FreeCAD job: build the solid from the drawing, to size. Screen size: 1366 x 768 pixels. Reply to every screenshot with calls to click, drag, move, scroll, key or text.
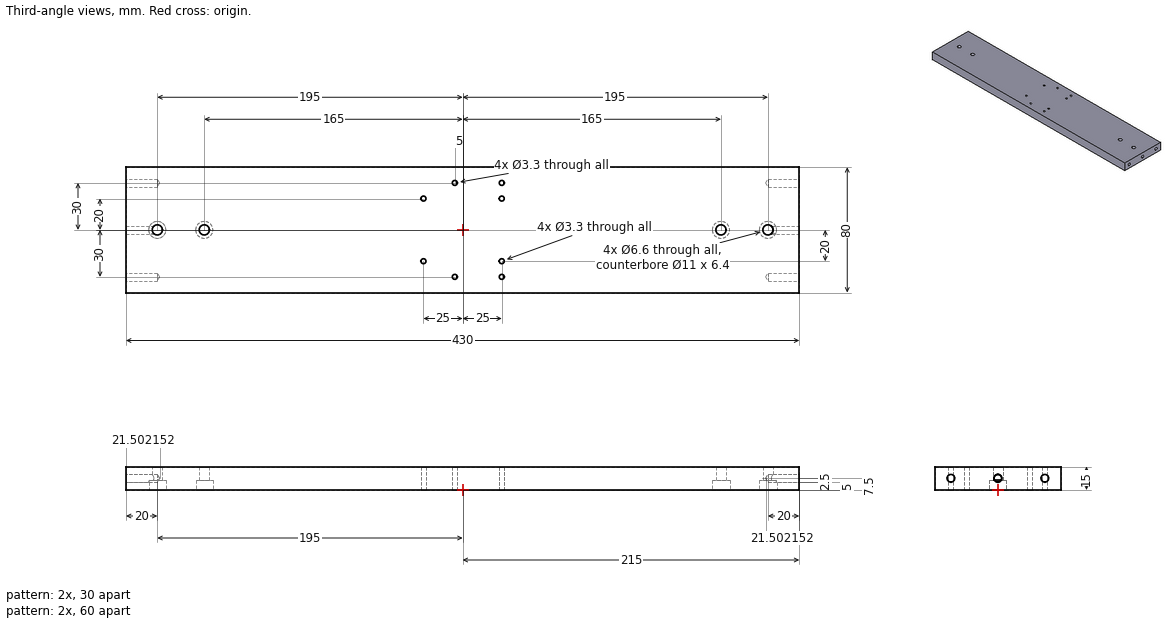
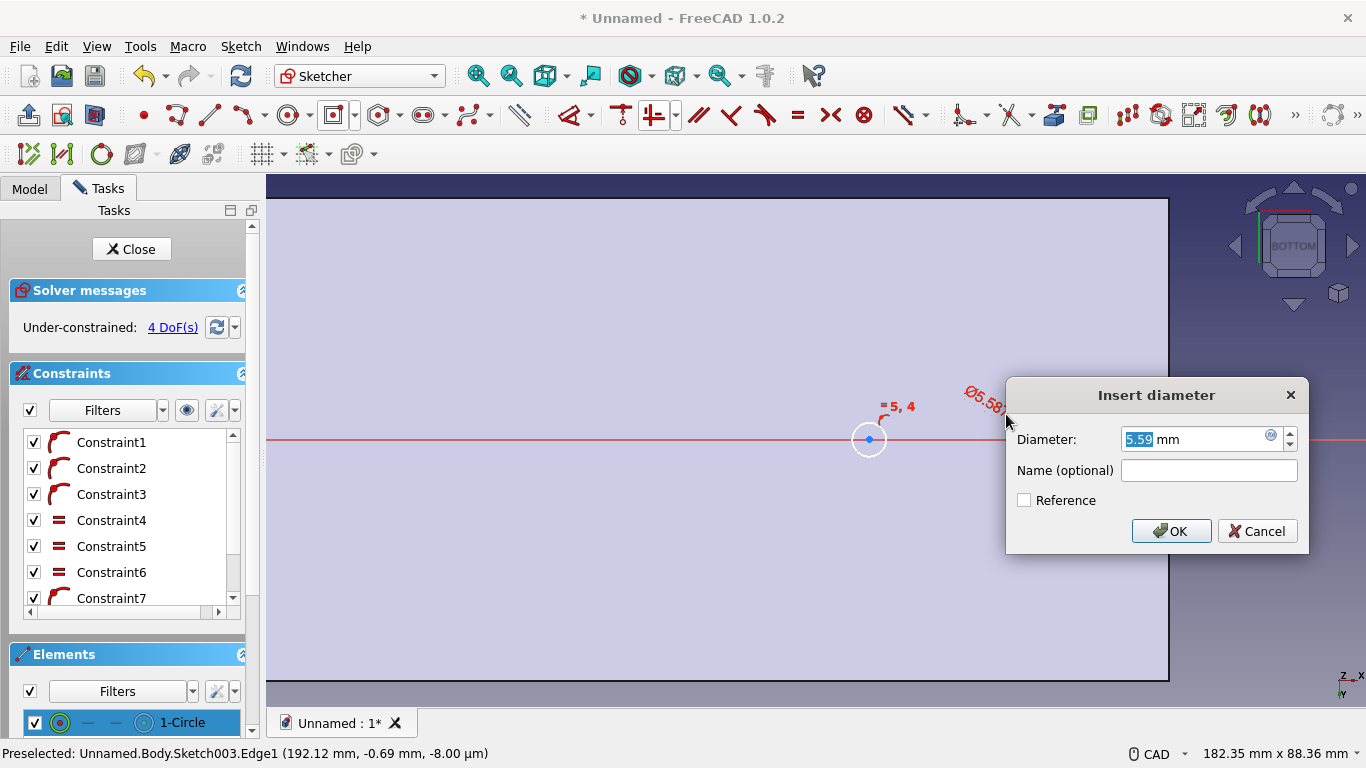
text(6.6)
key(Return)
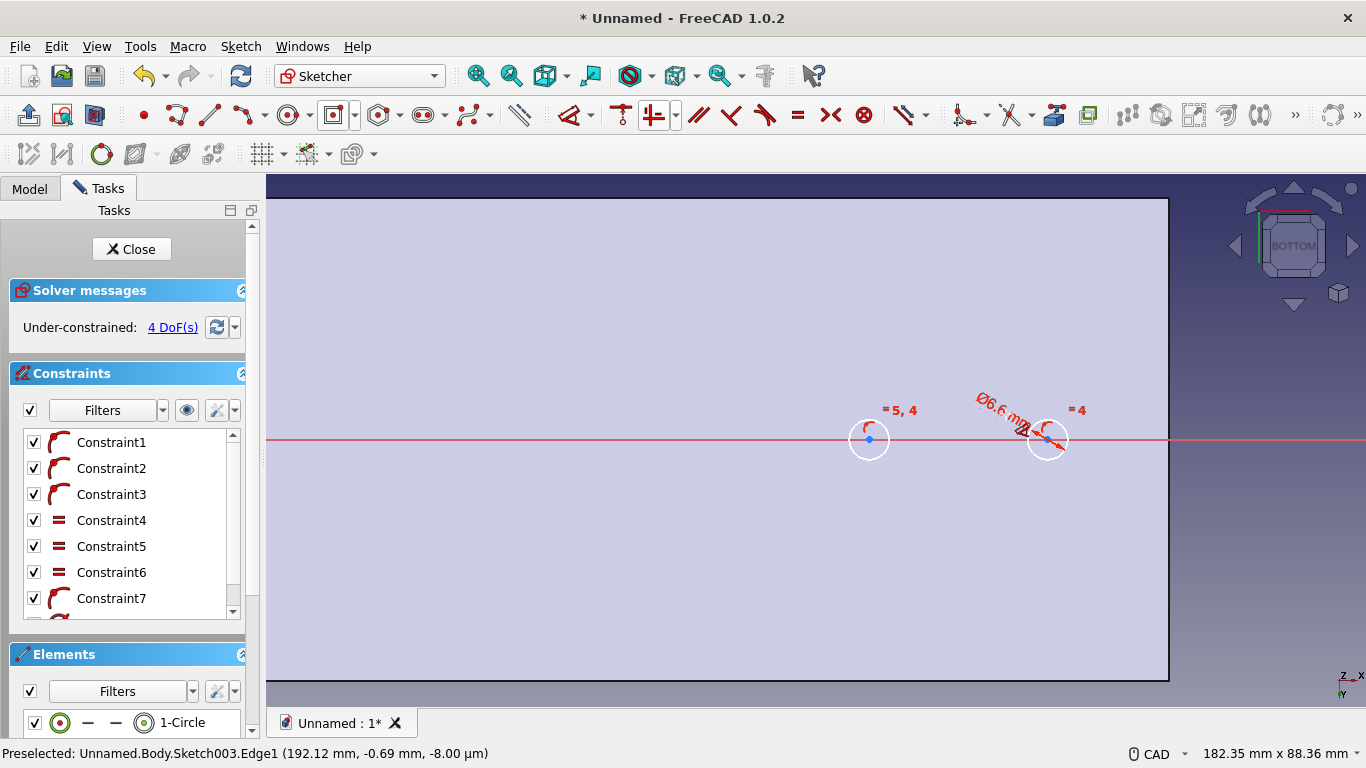
scroll(1034, 441, down, 7)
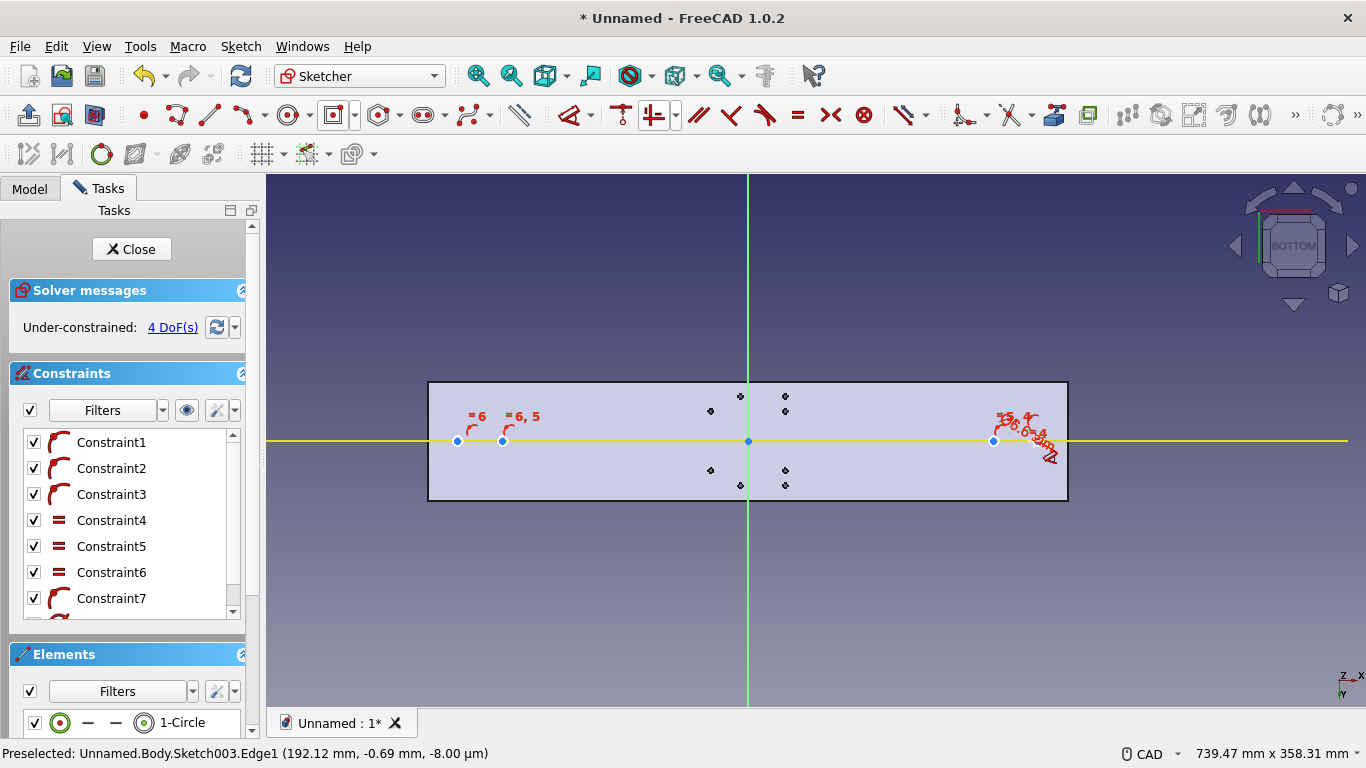
click(1038, 441)
click(893, 475)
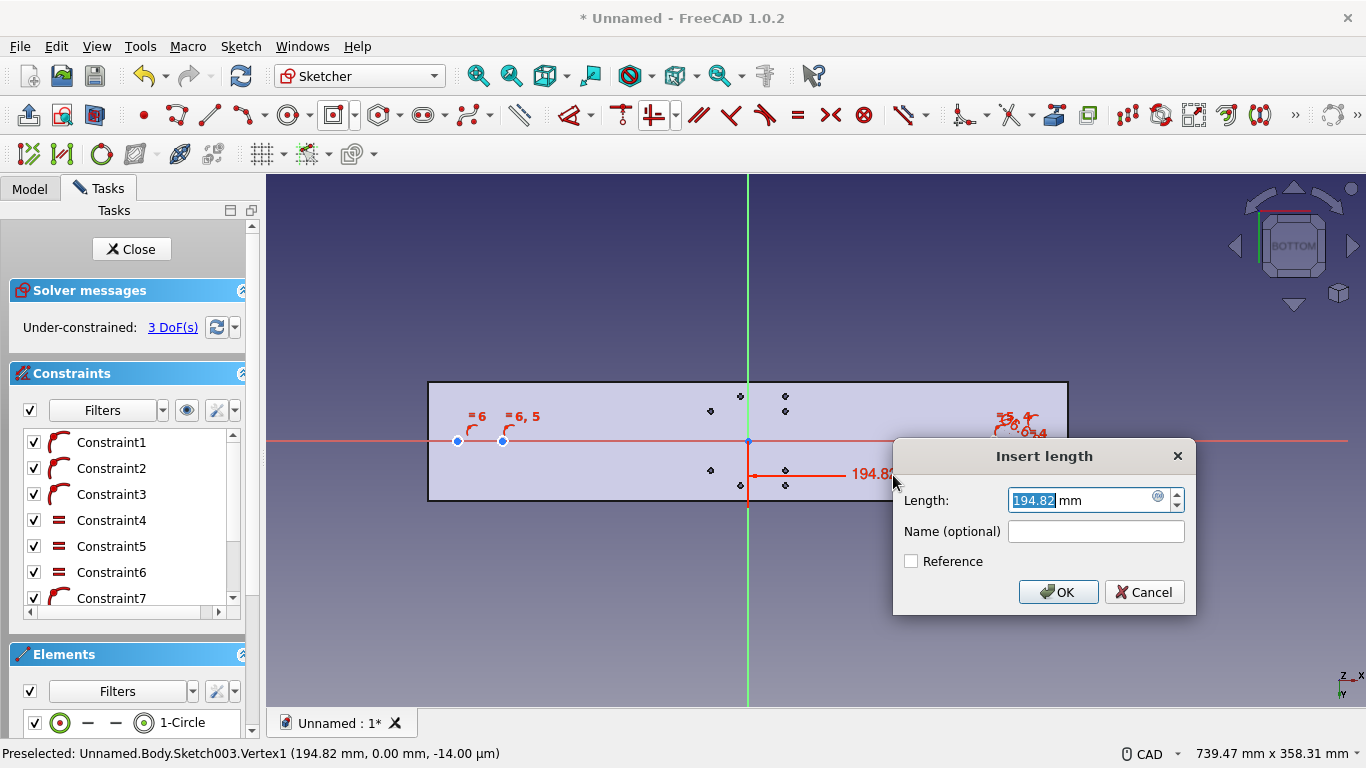
text(195)
key(Return)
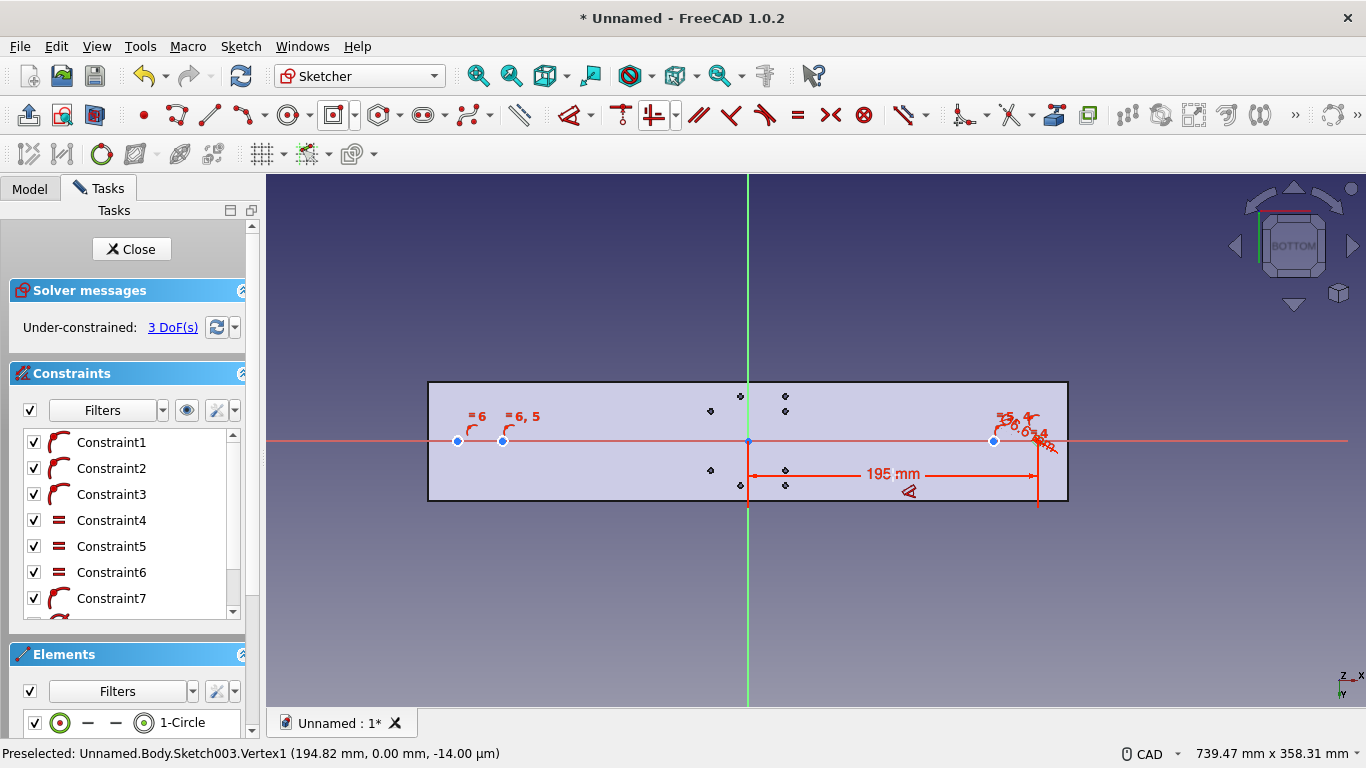
click(994, 441)
click(814, 475)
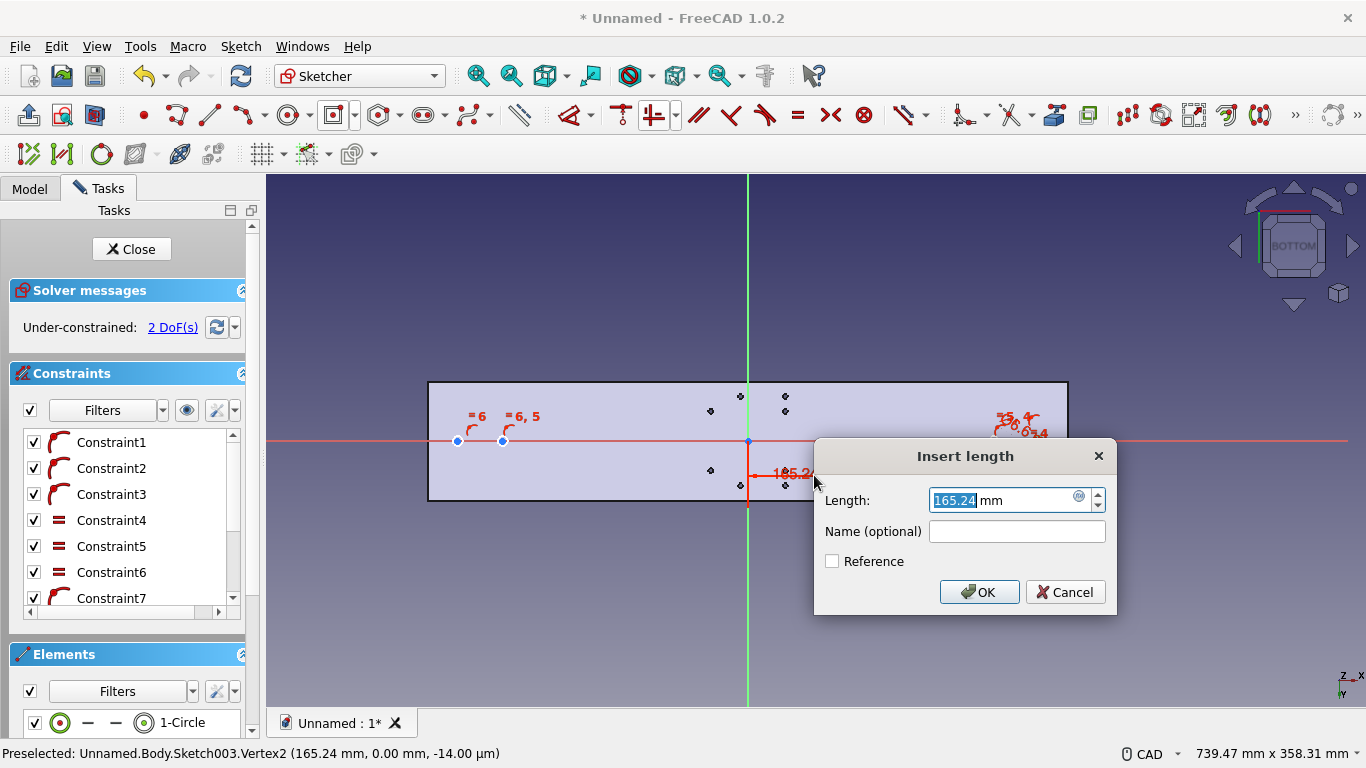
text(165)
key(Return)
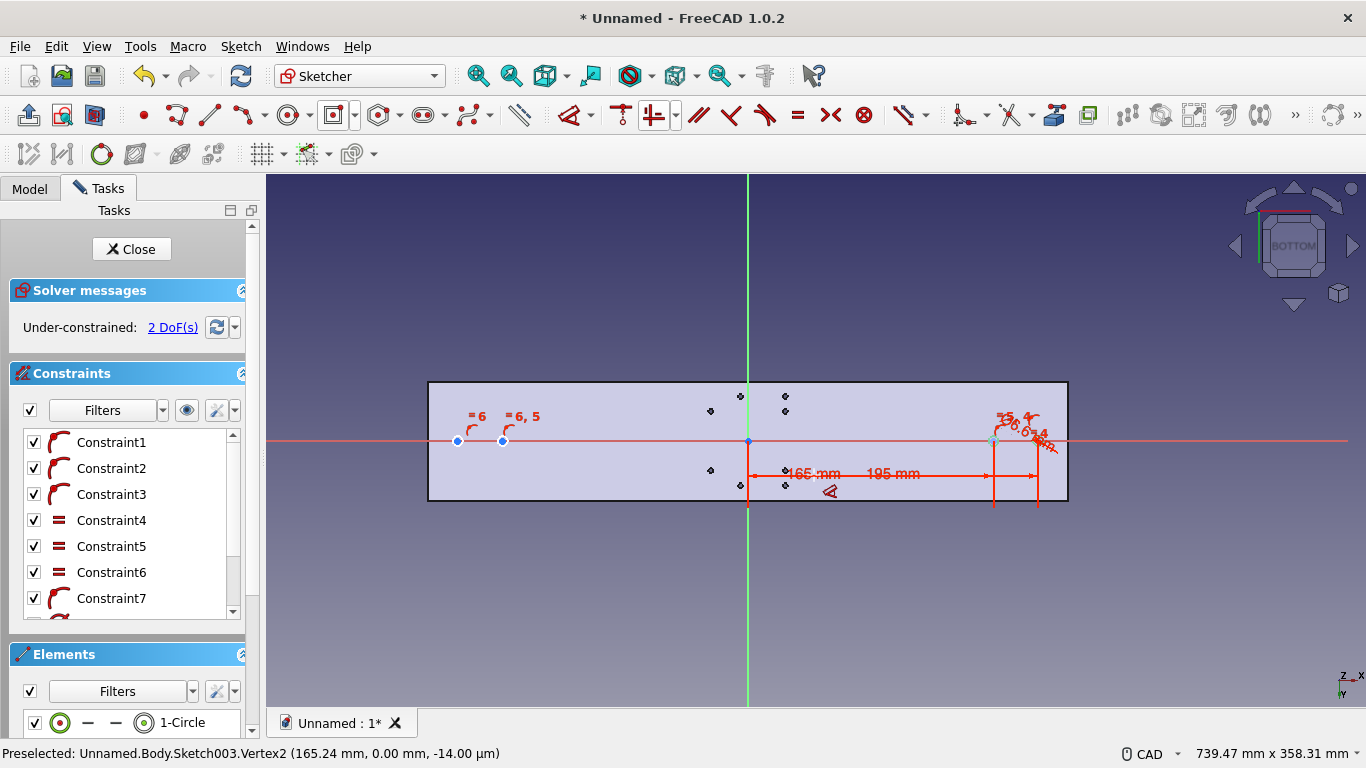
click(503, 441)
click(625, 475)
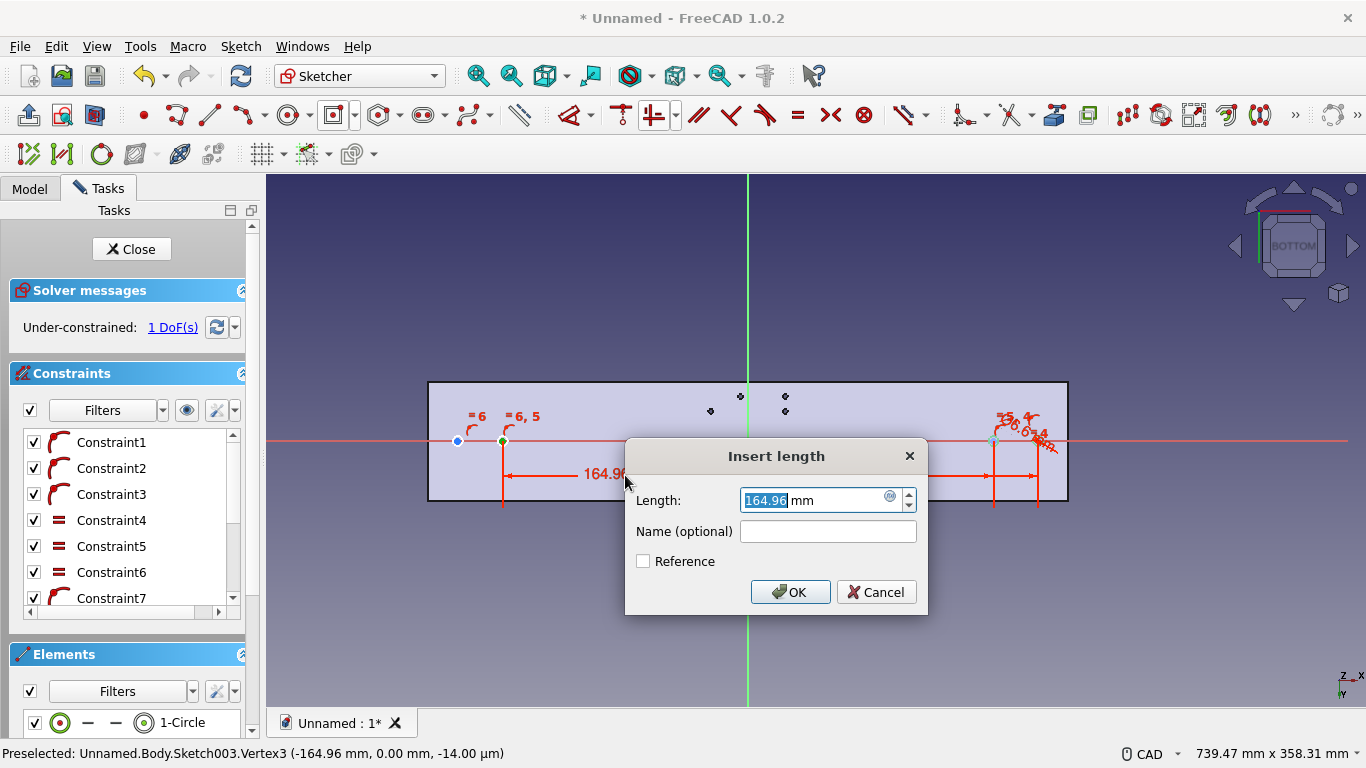
text(165)
key(Return)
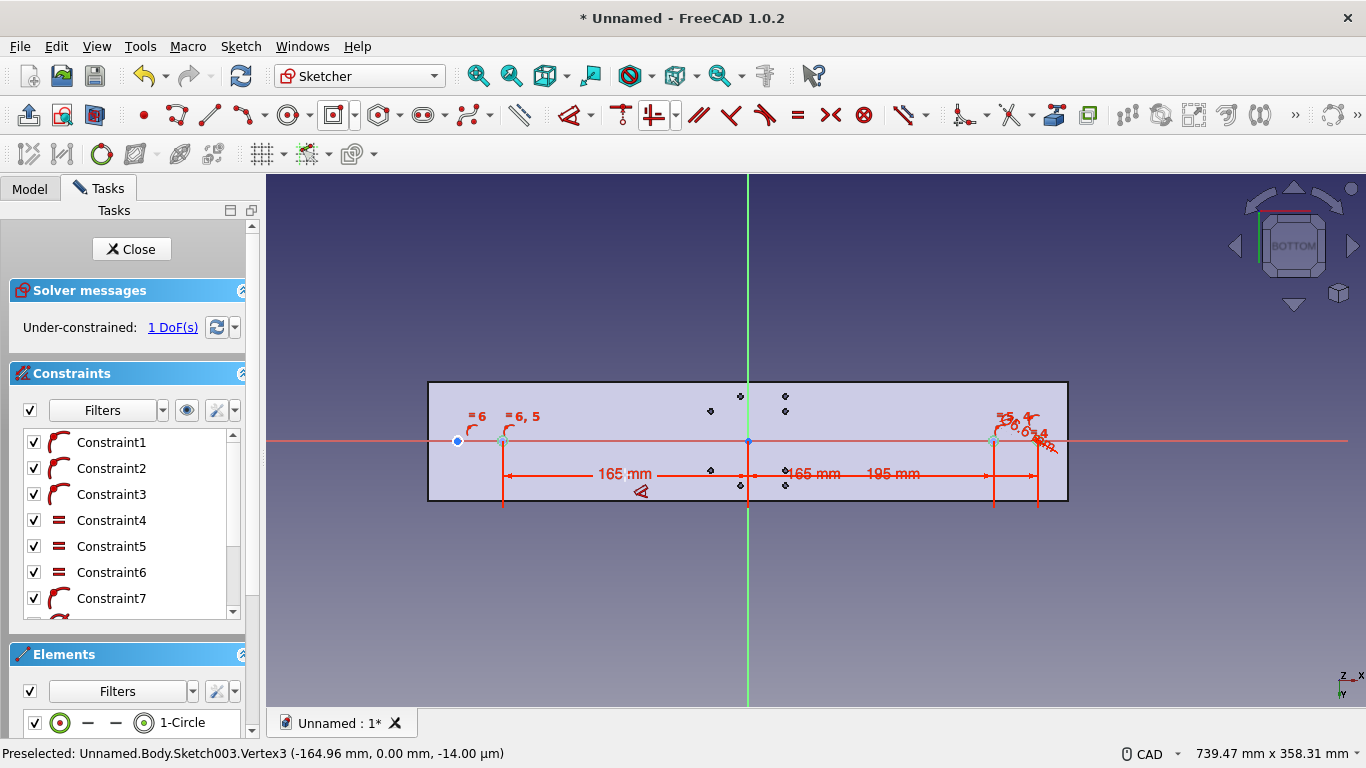
click(458, 441)
click(536, 475)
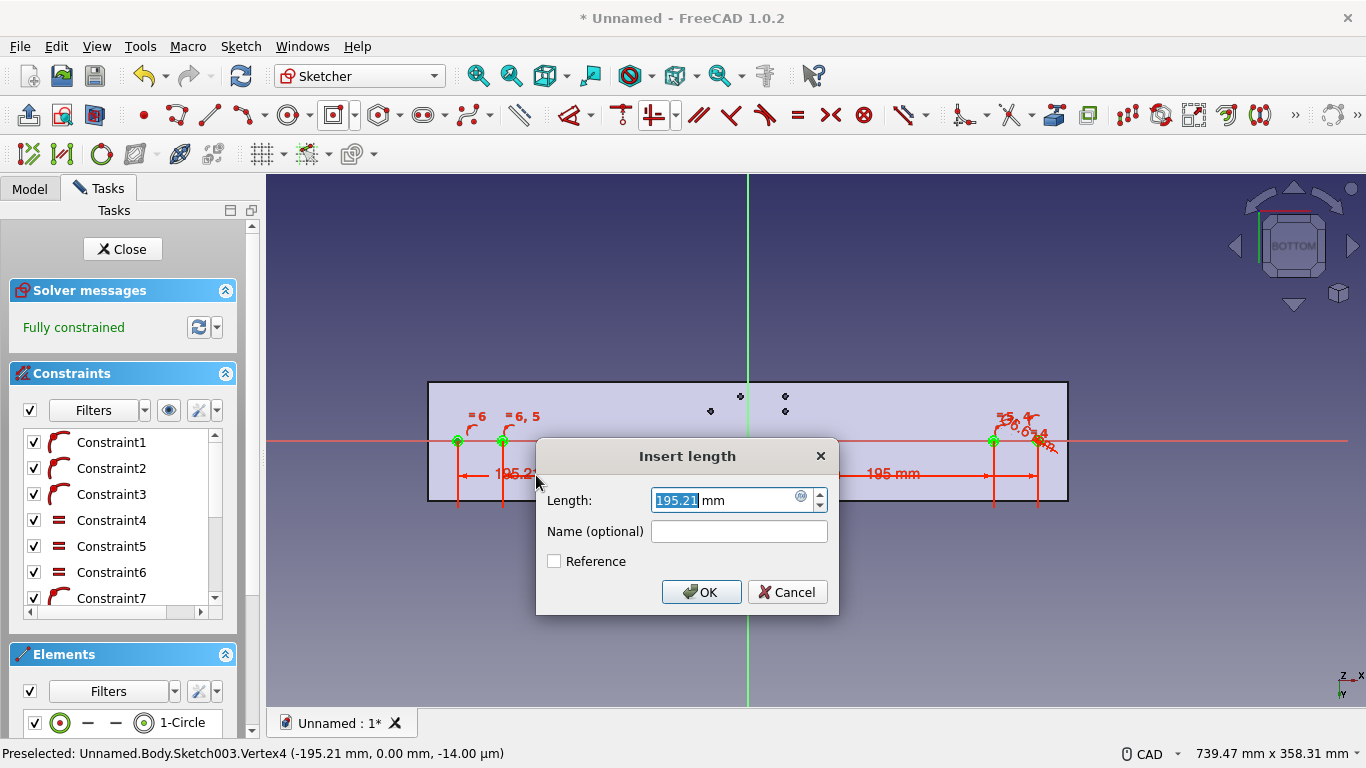
text(195)
key(Return)
key(Escape)